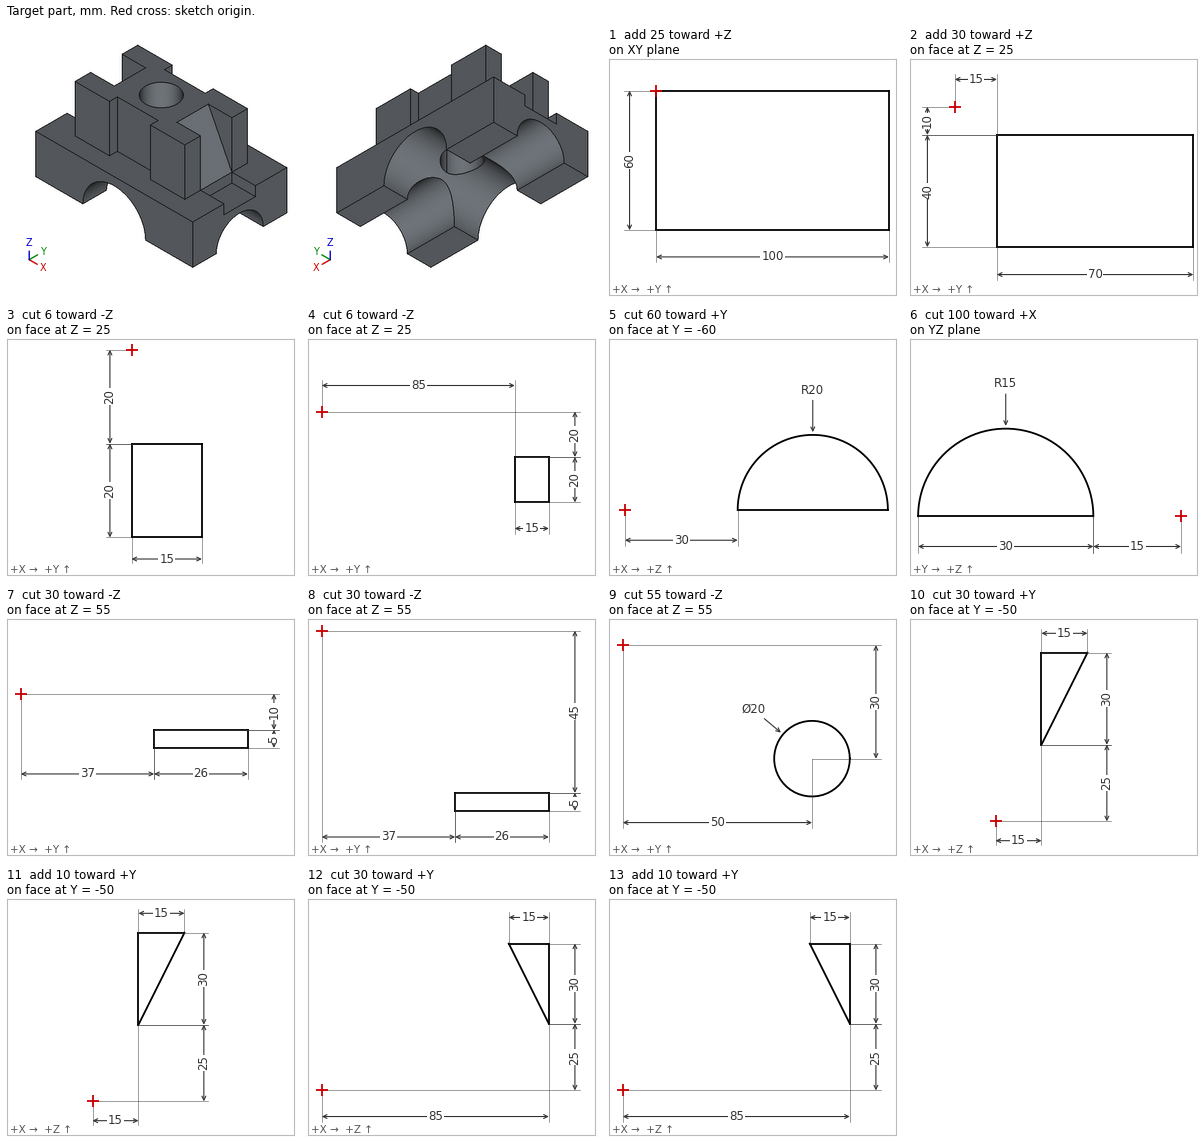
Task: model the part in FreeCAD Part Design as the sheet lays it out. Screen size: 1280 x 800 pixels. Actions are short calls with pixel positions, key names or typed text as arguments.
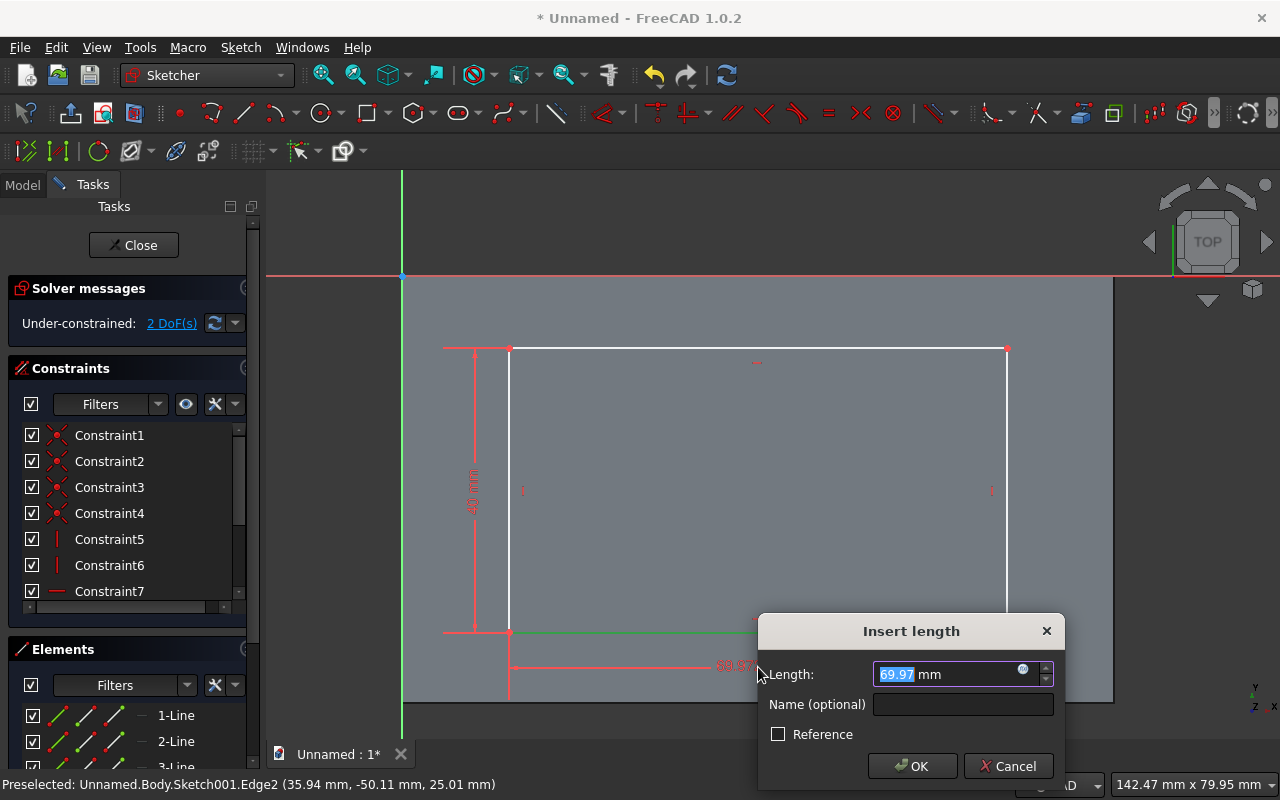
text(70)
key(Return)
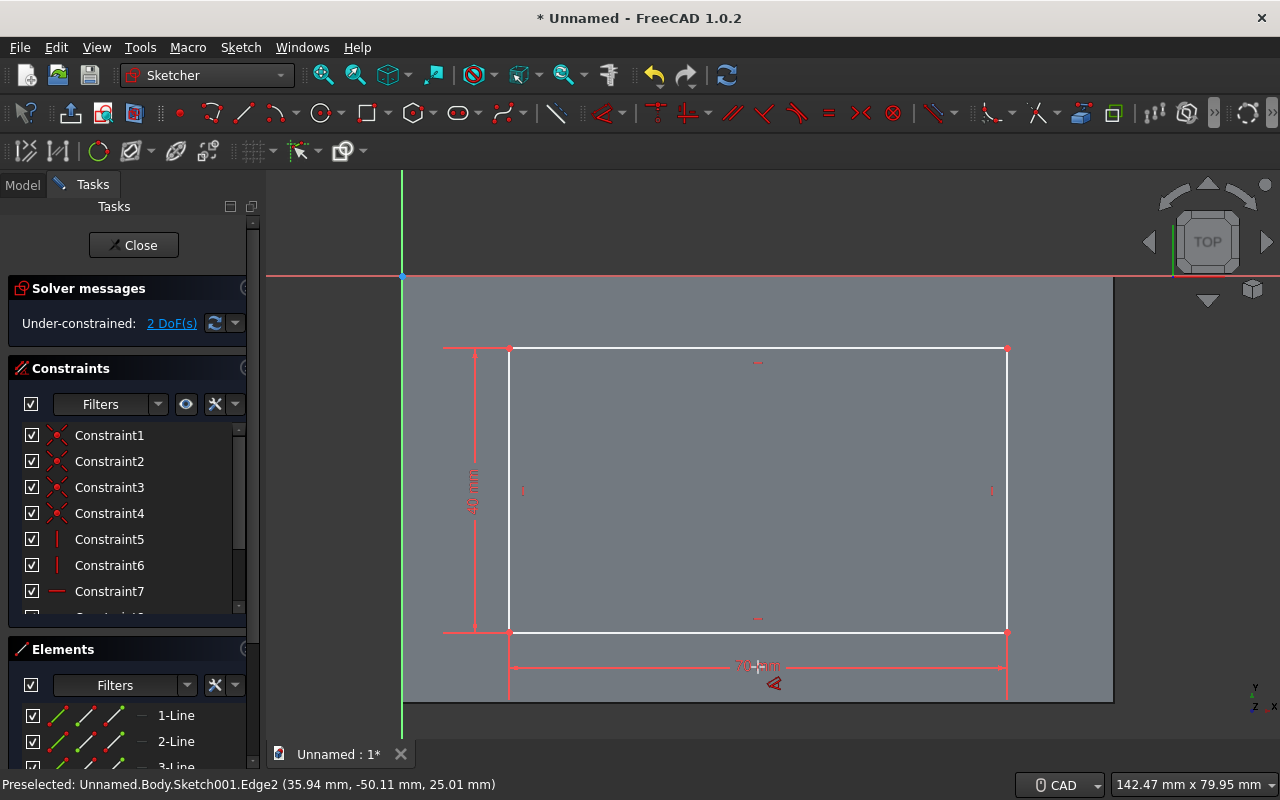
click(509, 348)
click(456, 242)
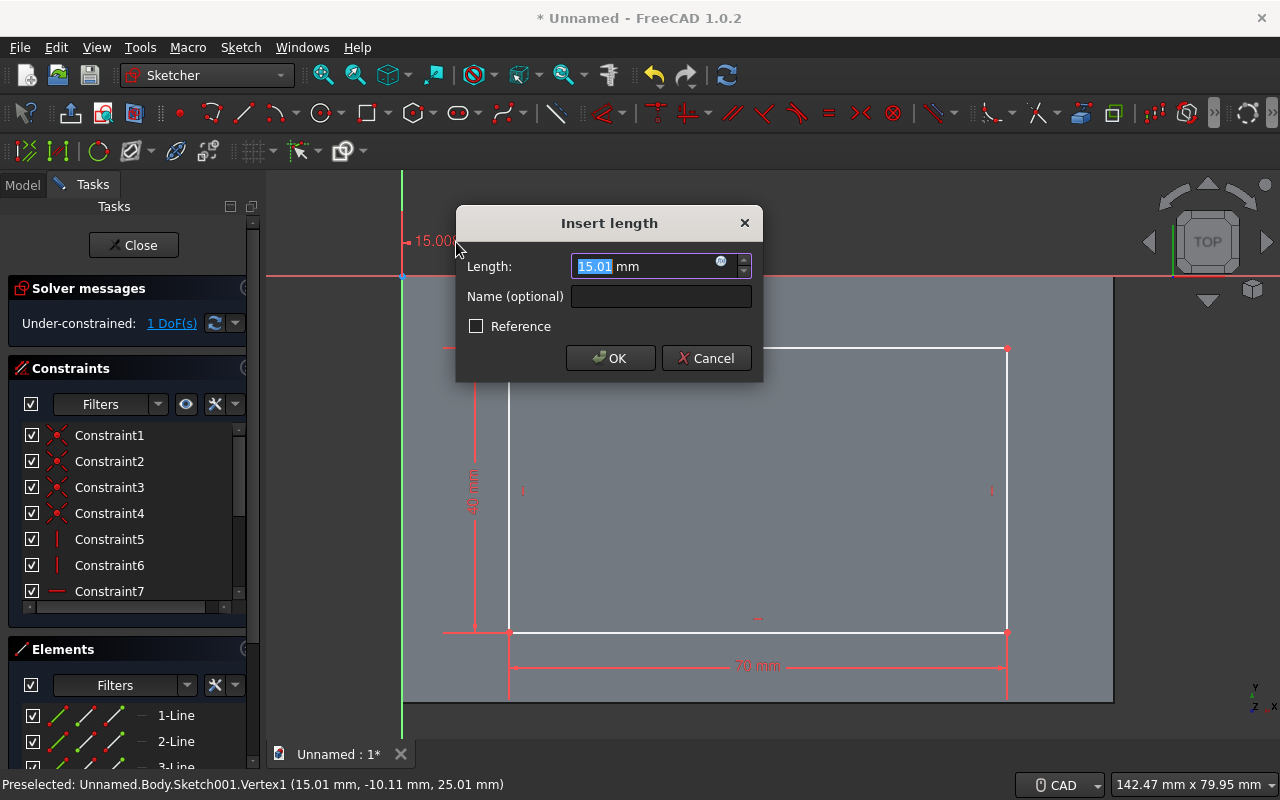
text(15)
key(Return)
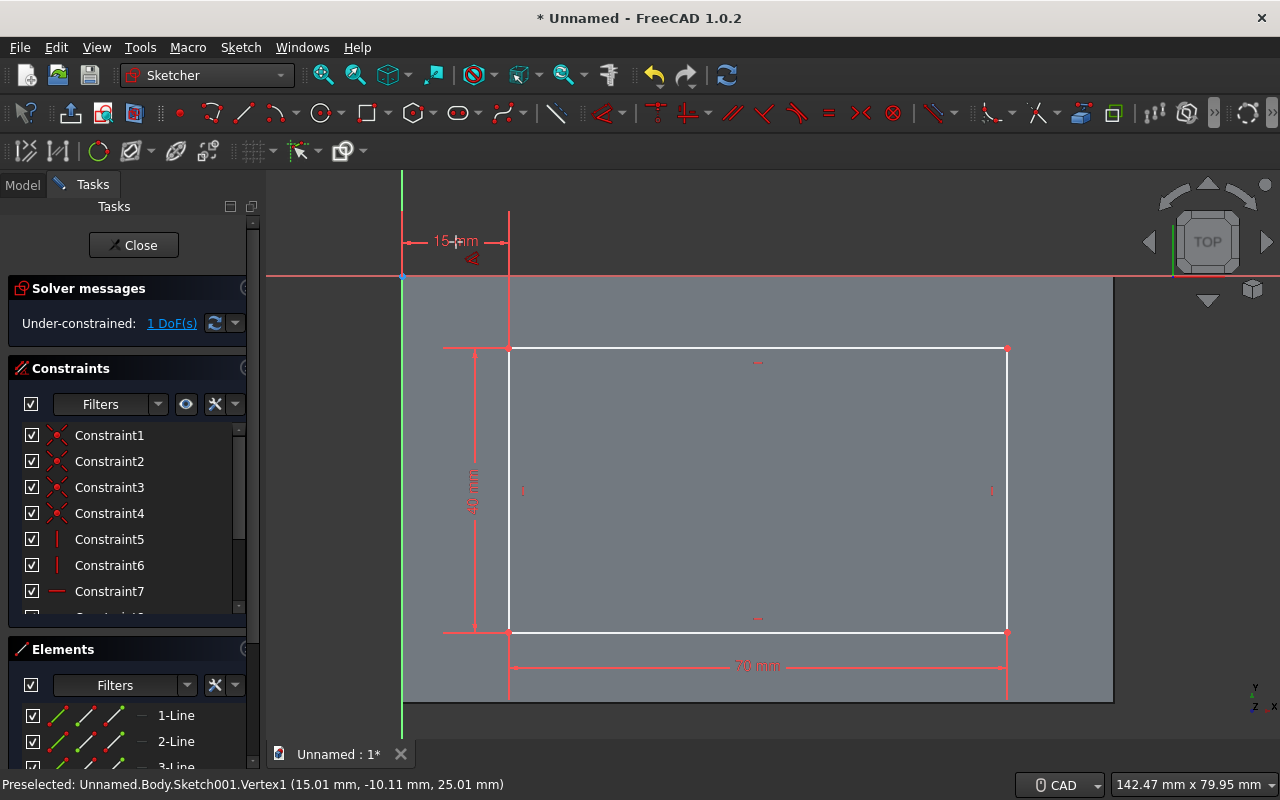
click(509, 348)
click(368, 312)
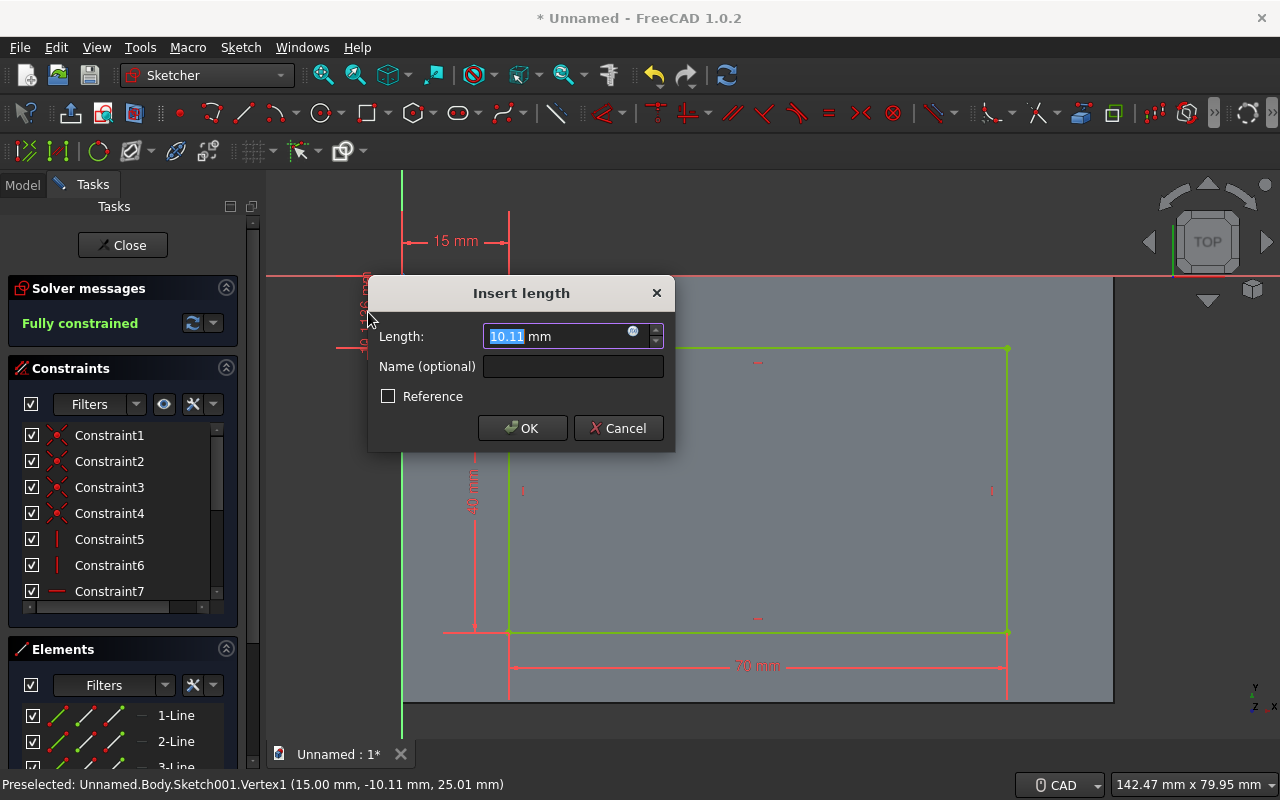
text(10)
key(Return)
key(Escape)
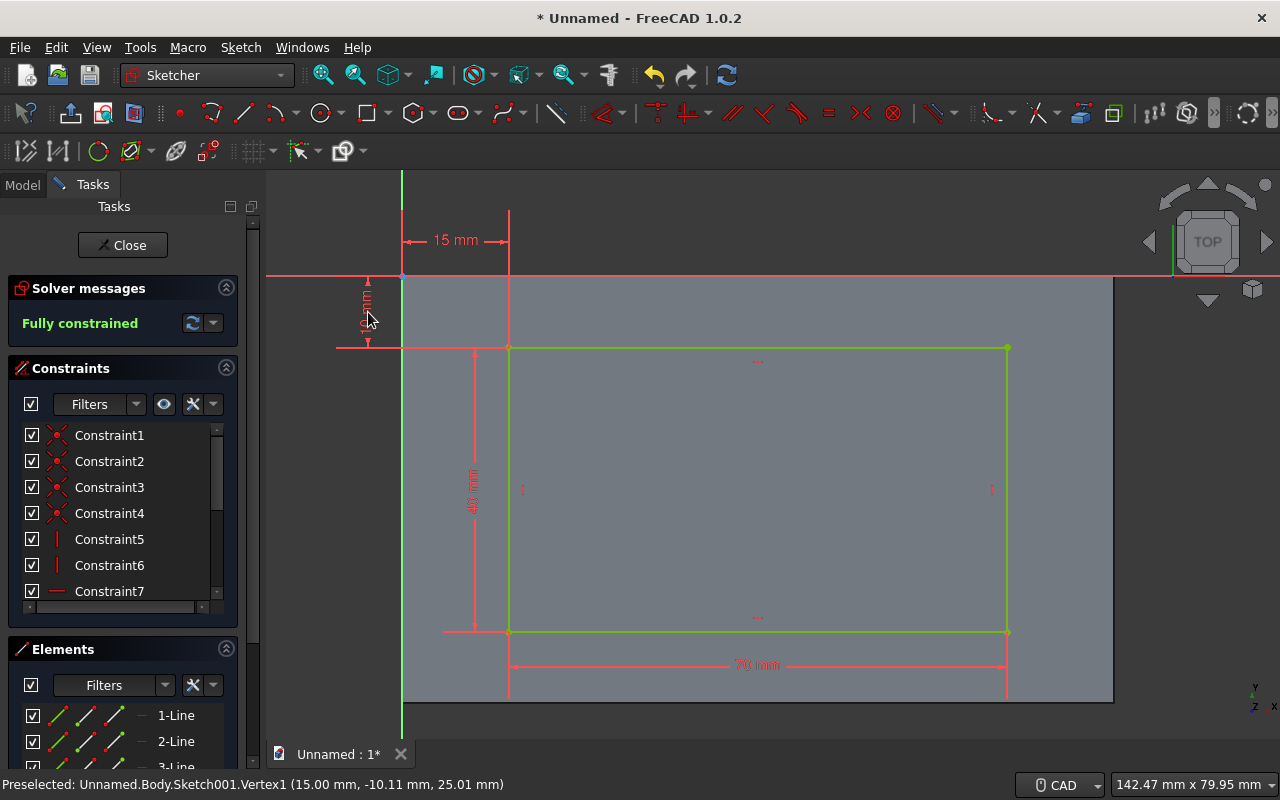
click(123, 245)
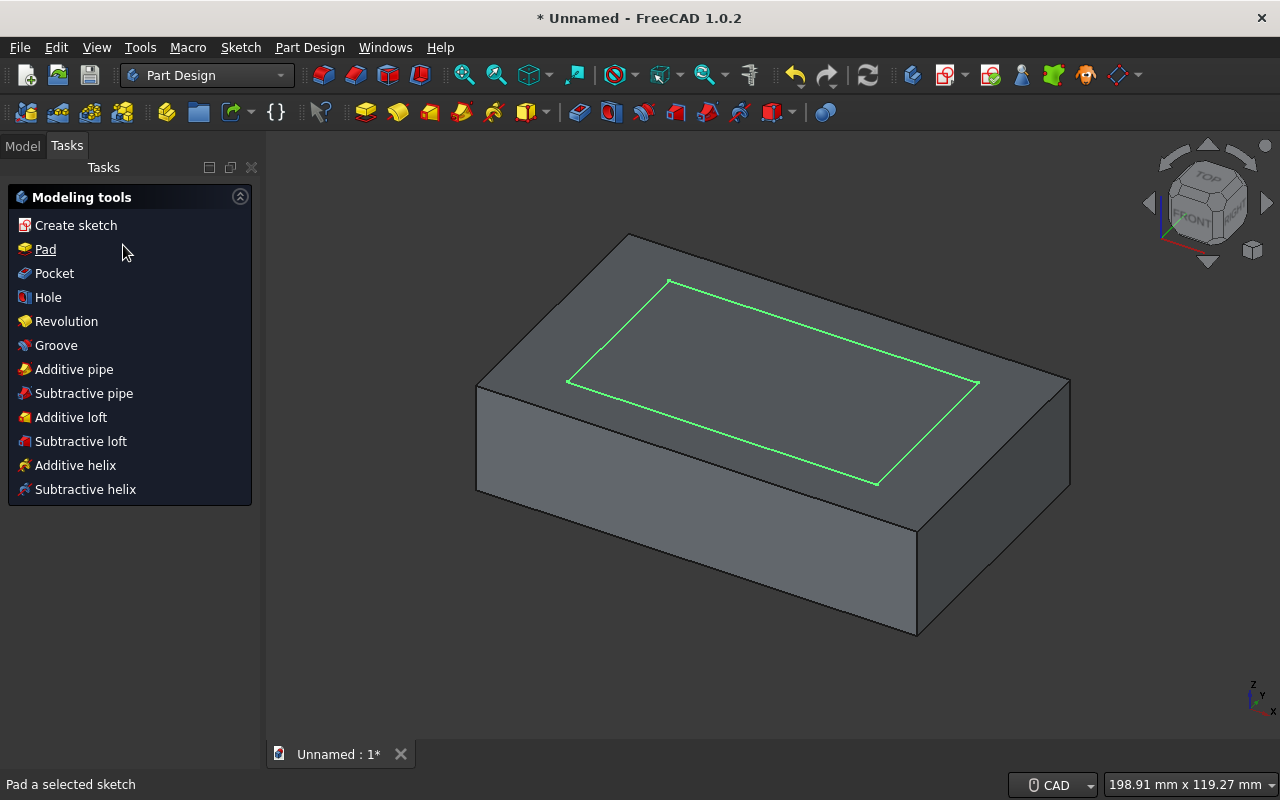
click(366, 112)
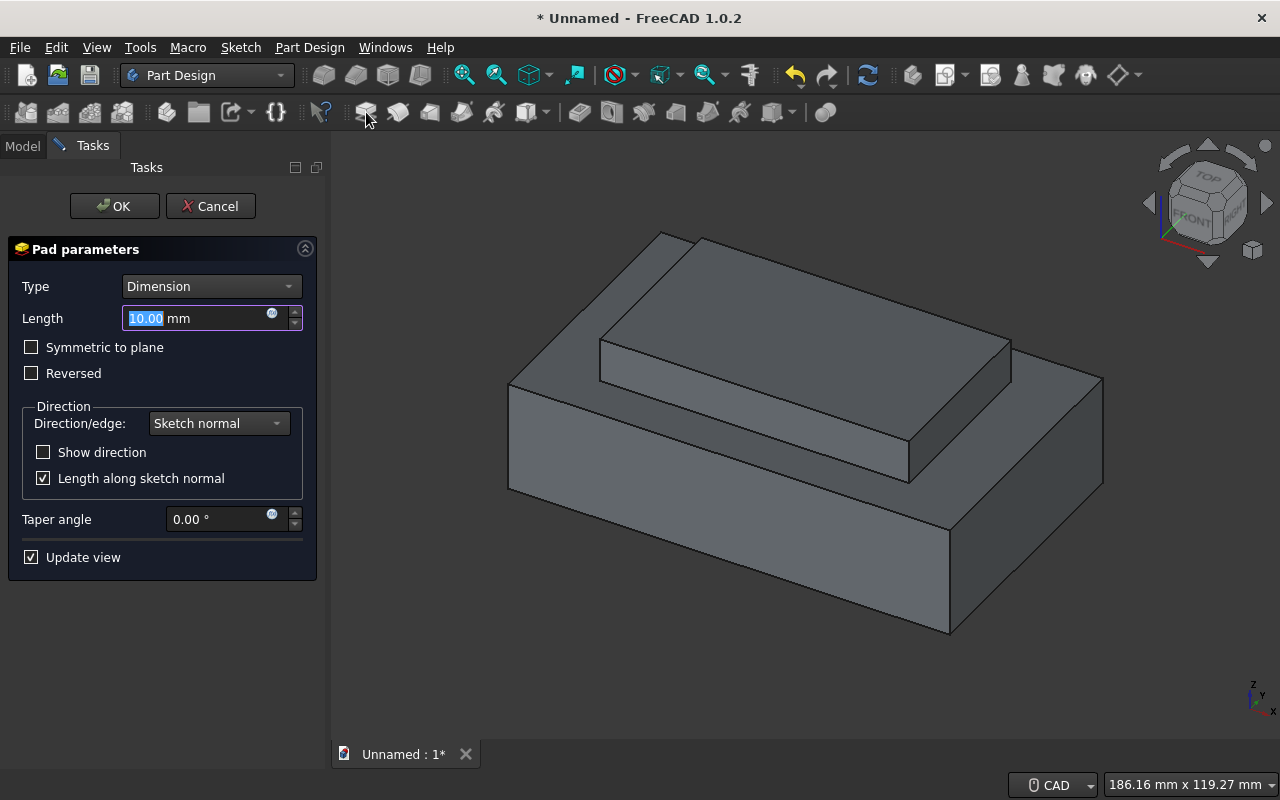
text(30)
key(Tab)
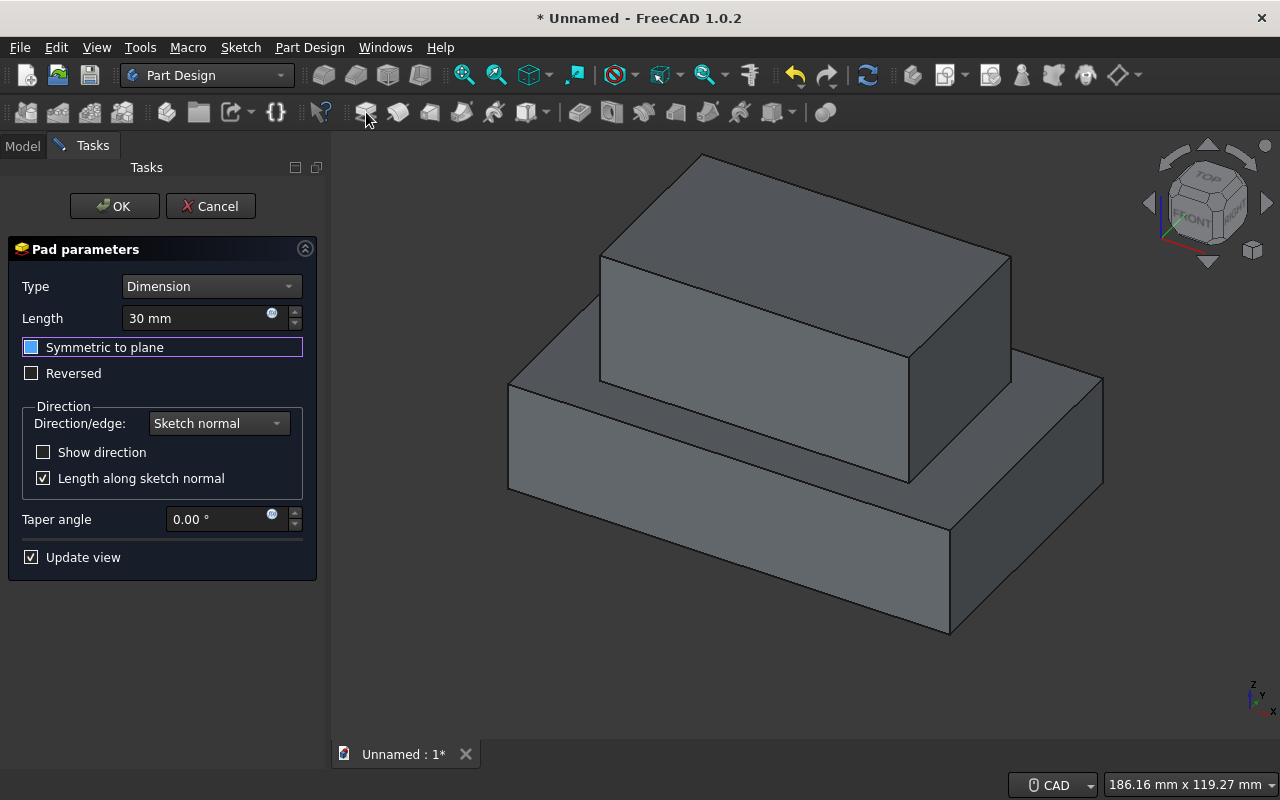
click(115, 206)